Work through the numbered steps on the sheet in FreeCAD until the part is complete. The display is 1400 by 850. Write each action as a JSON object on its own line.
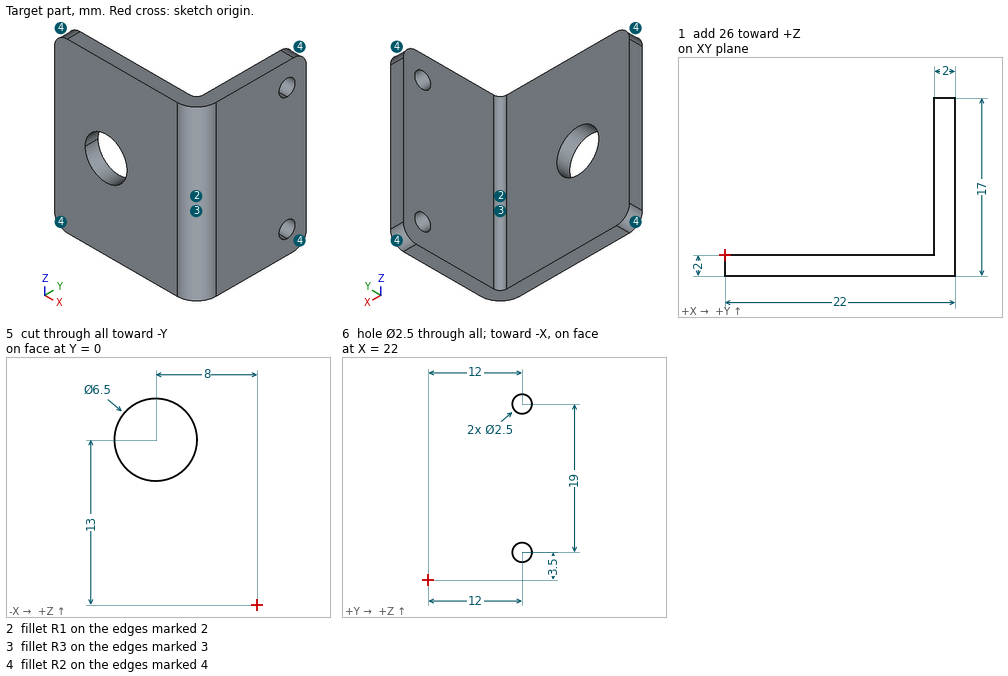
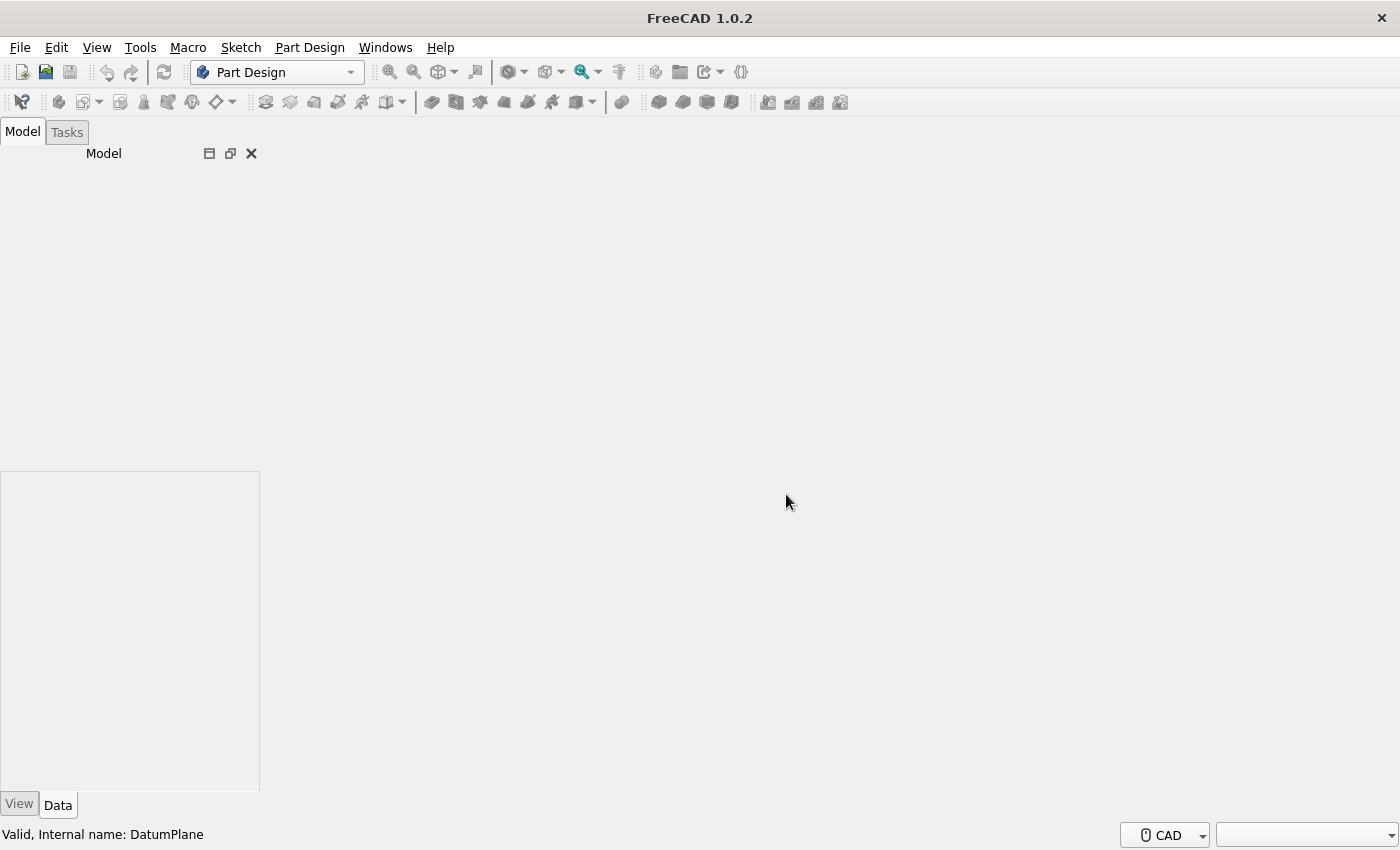
{"action": "left_click", "coordinate": [22, 72]}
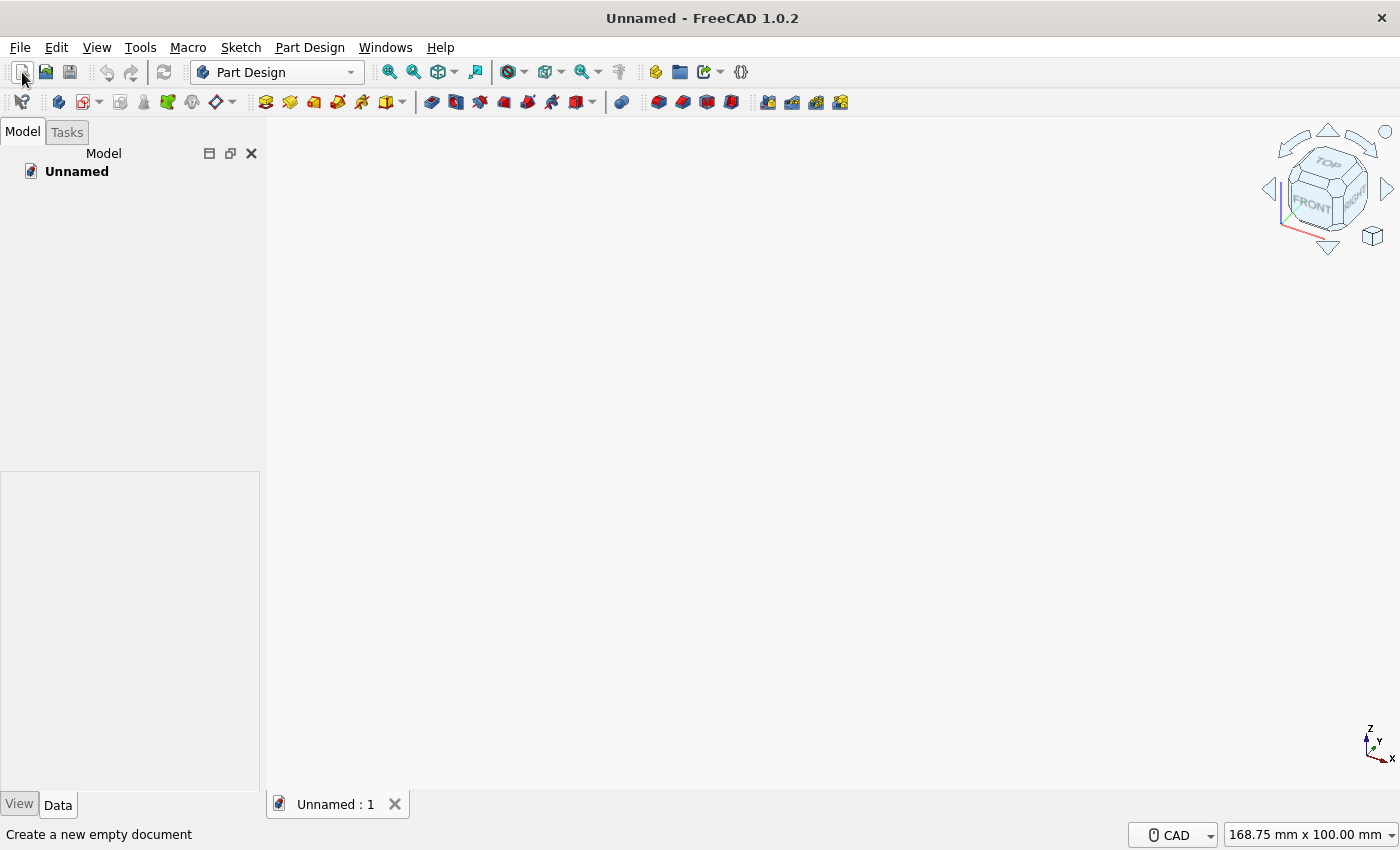
{"action": "left_click", "coordinate": [84, 102]}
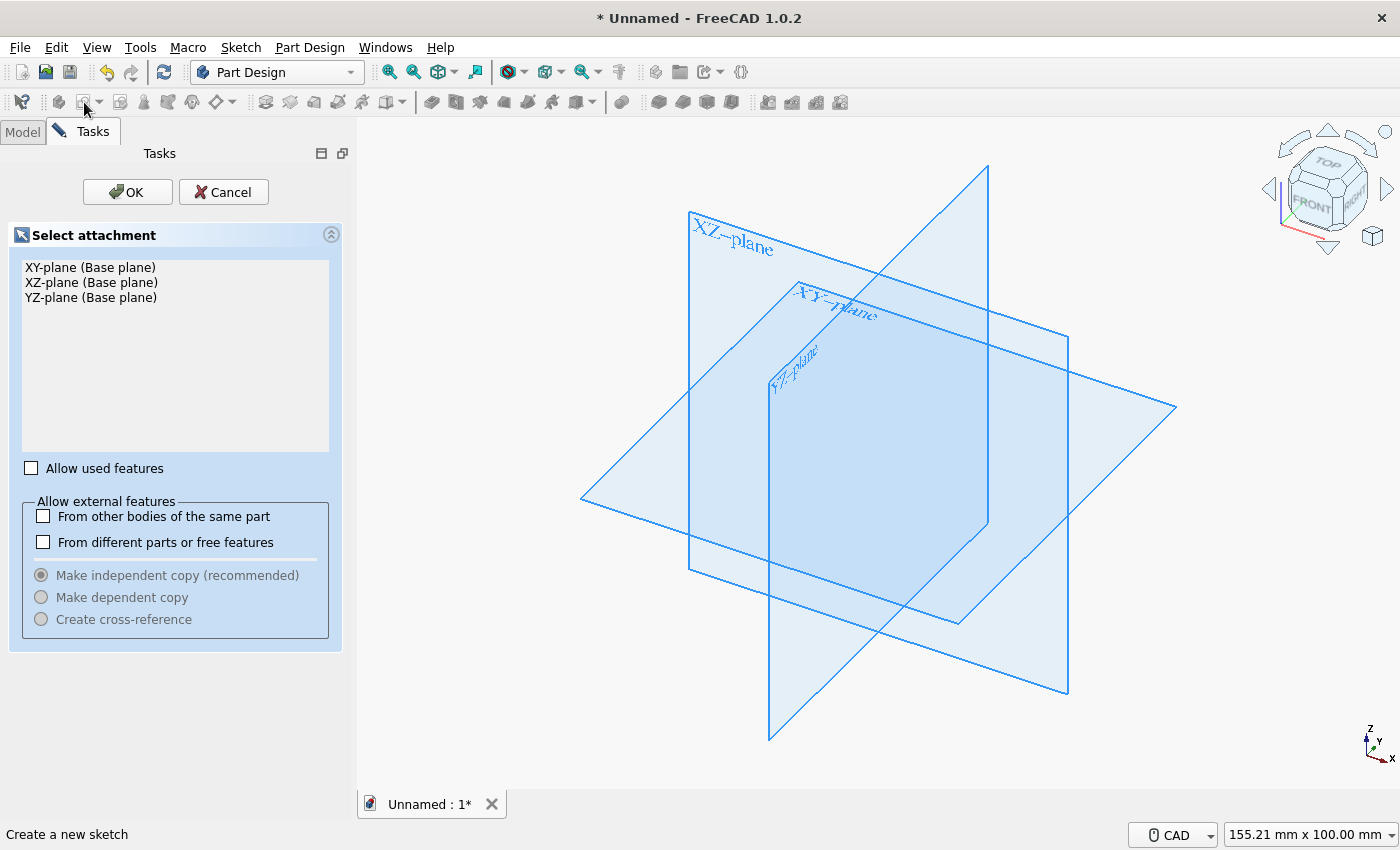
{"action": "left_click", "coordinate": [82, 268]}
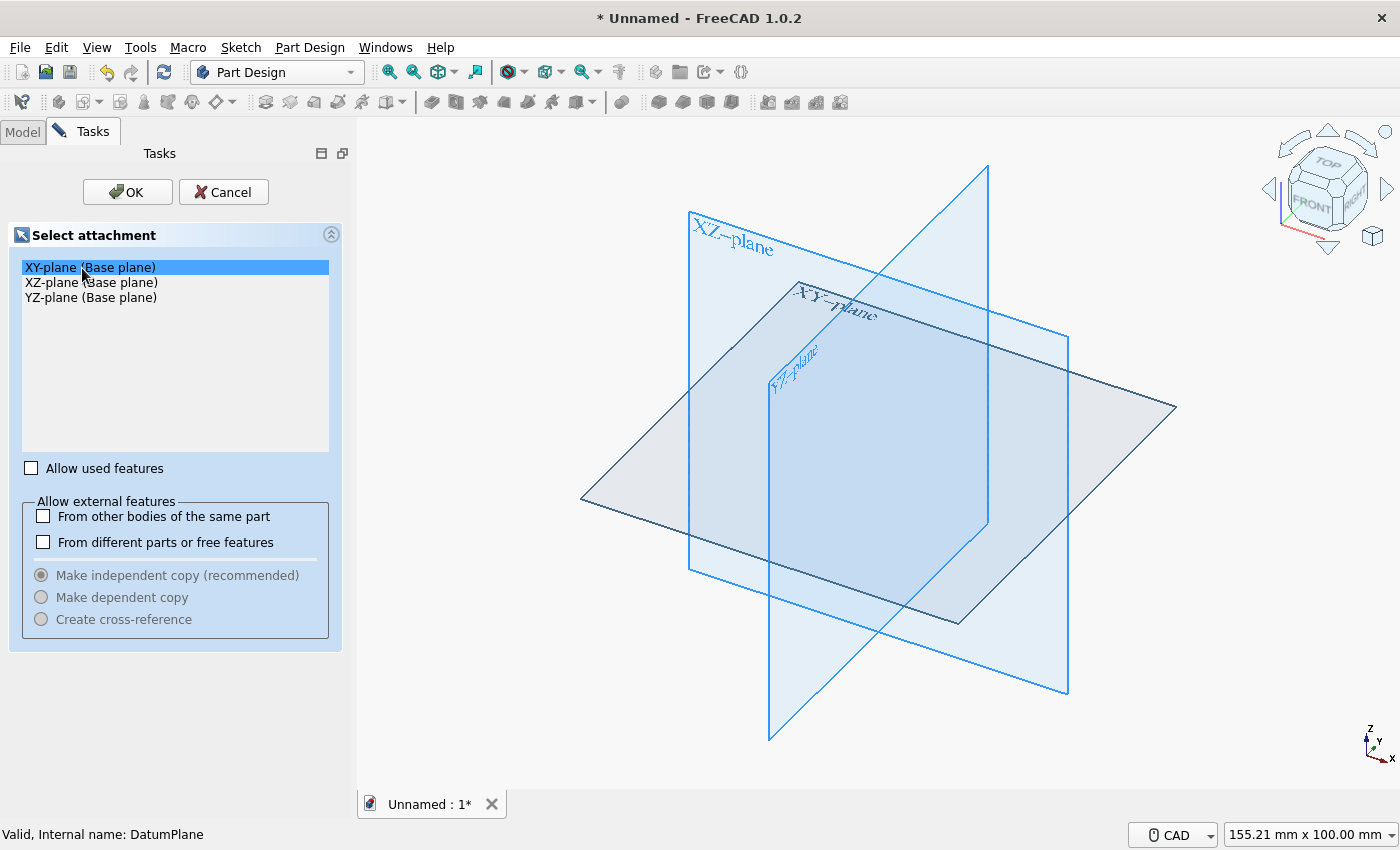
{"action": "left_click", "coordinate": [128, 192]}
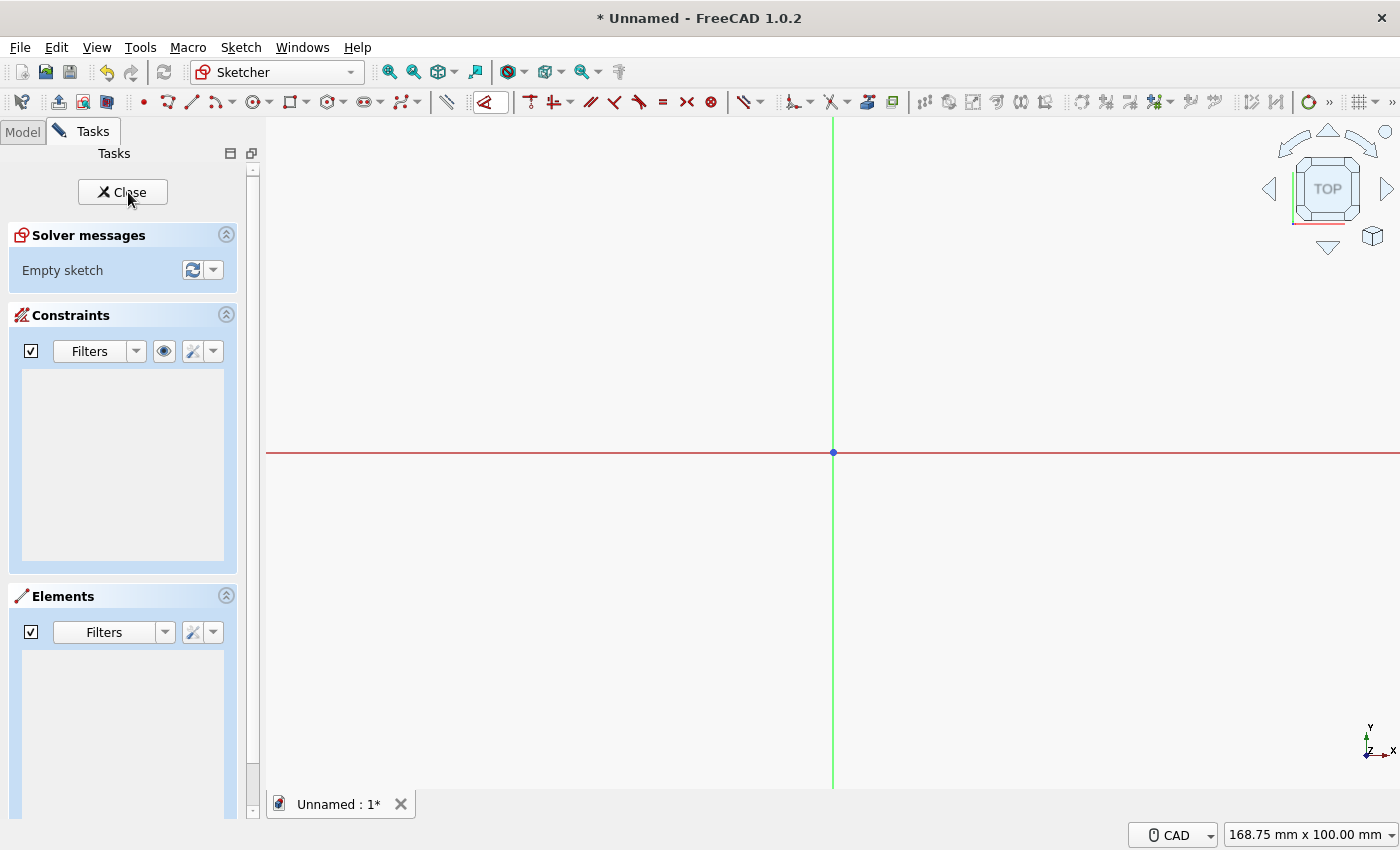
{"action": "scroll", "coordinate": [954, 395], "scroll_direction": "up", "scroll_amount": 7}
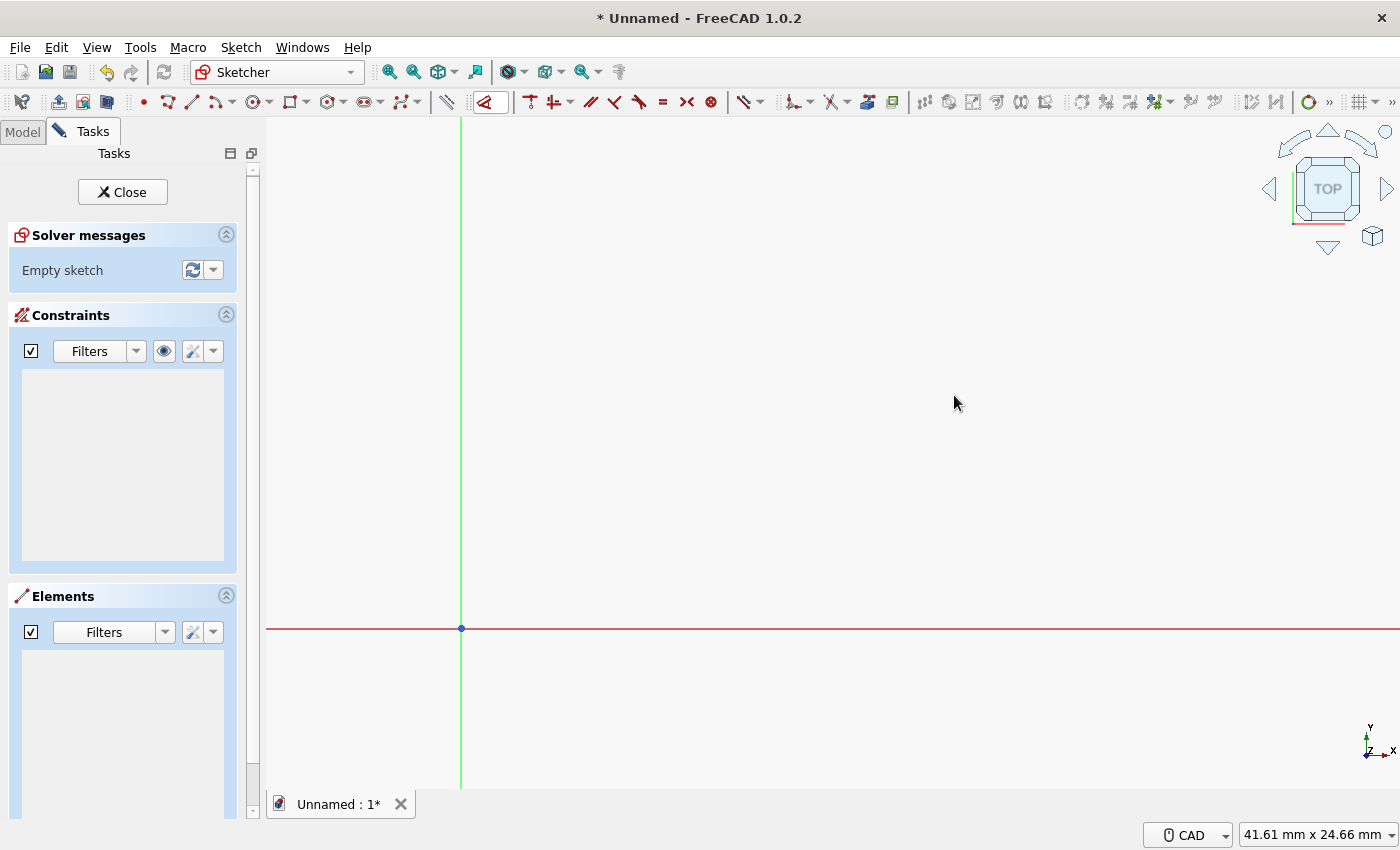
{"action": "key", "text": "g m"}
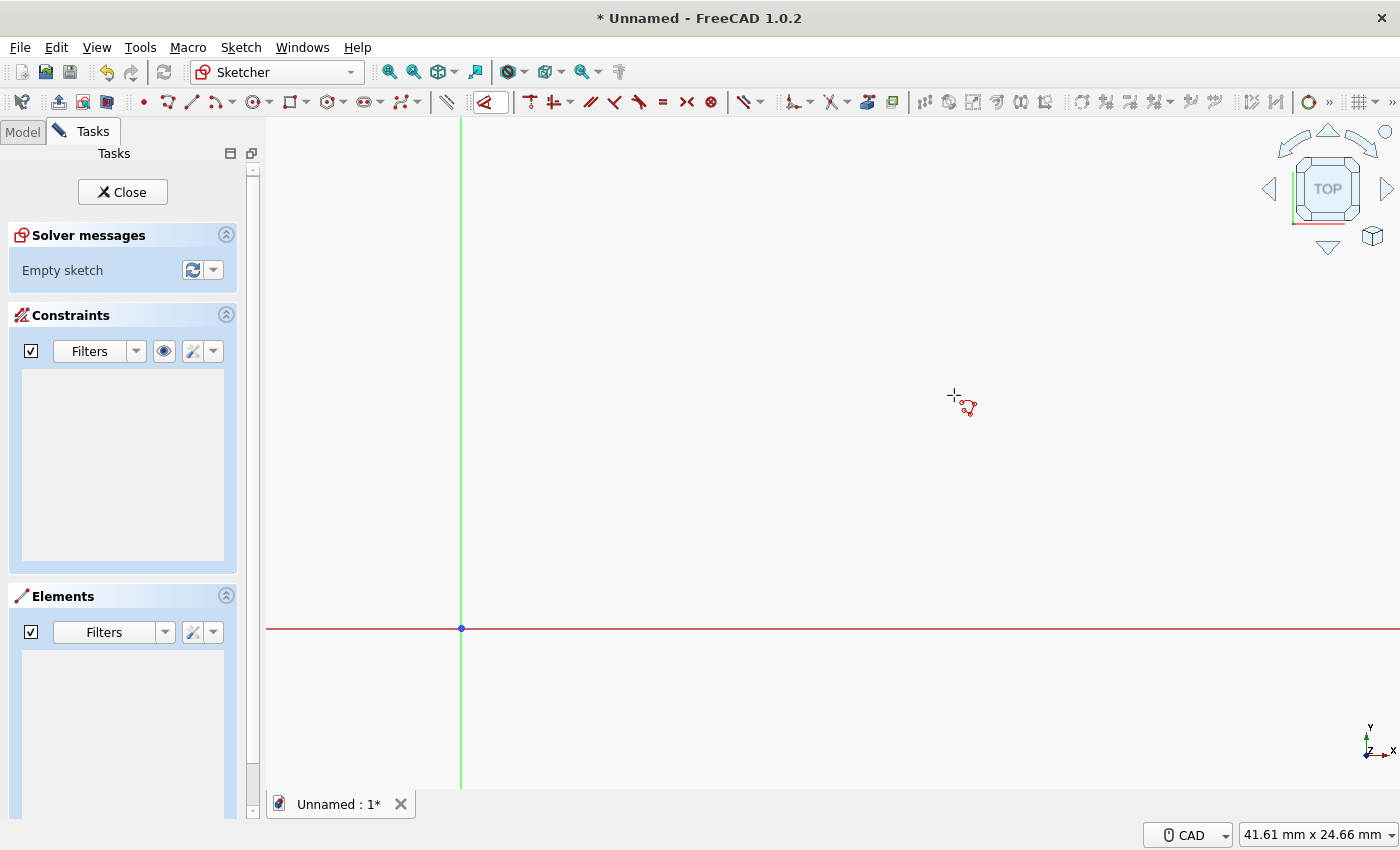
{"action": "left_click", "coordinate": [461, 629]}
{"action": "left_click", "coordinate": [470, 683]}
{"action": "left_click", "coordinate": [1061, 683]}
{"action": "left_click", "coordinate": [1061, 220]}
{"action": "left_click", "coordinate": [1006, 220]}
{"action": "left_click", "coordinate": [1006, 620]}
{"action": "left_click", "coordinate": [461, 629]}
{"action": "key", "text": "Escape"}
{"action": "key", "text": "Escape"}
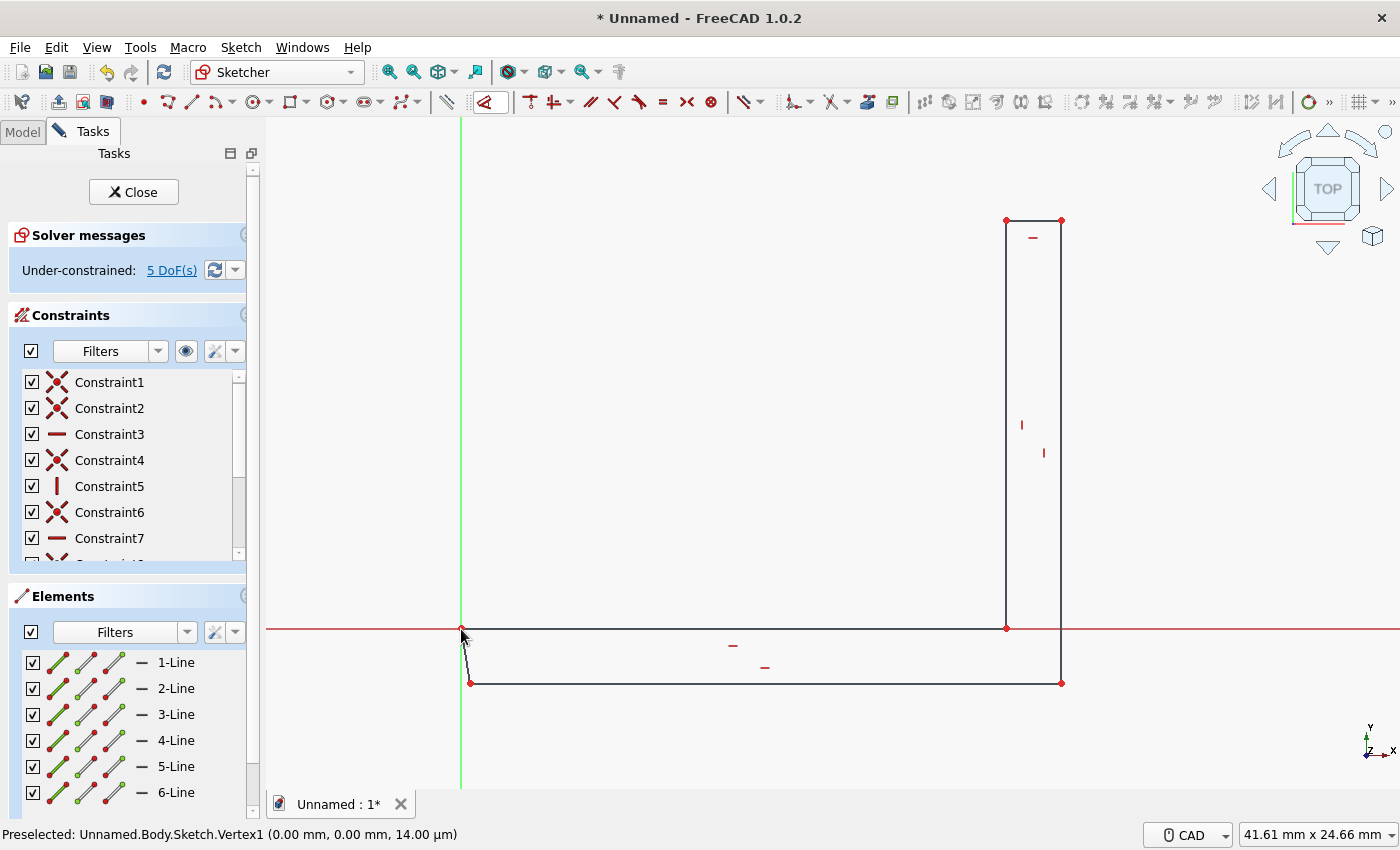
{"action": "left_click", "coordinate": [464, 645]}